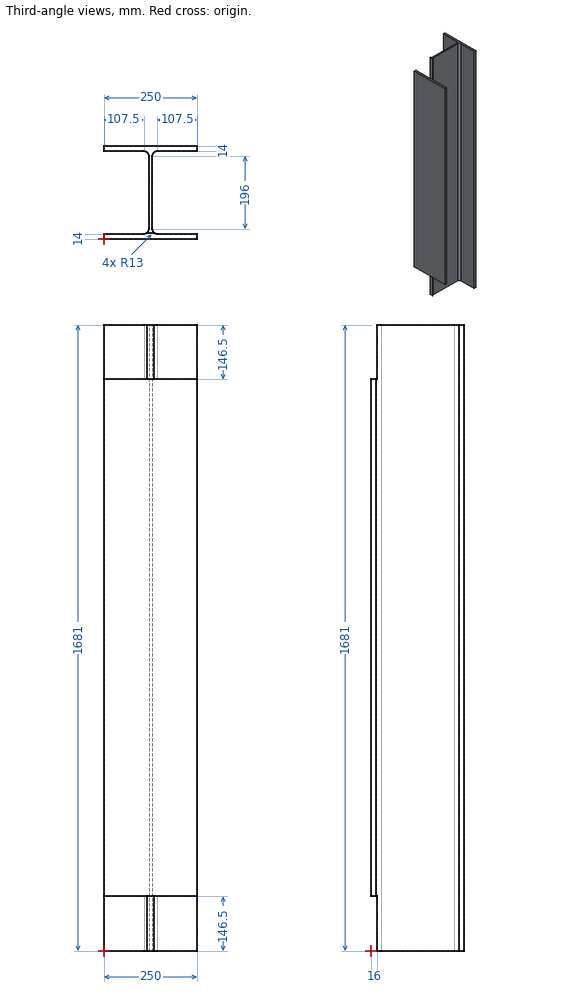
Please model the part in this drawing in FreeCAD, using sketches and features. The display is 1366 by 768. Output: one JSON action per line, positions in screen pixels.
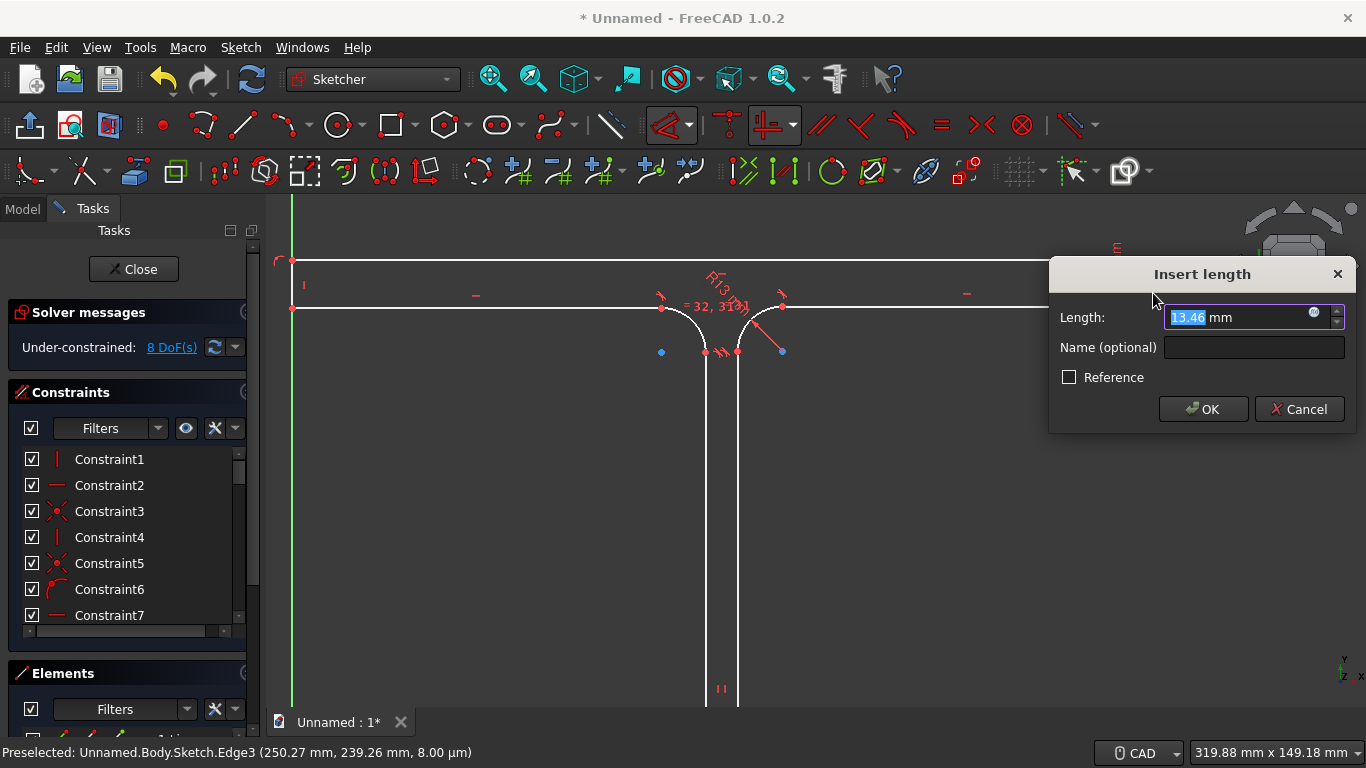
{"action": "type", "text": "14"}
{"action": "key", "text": "Return"}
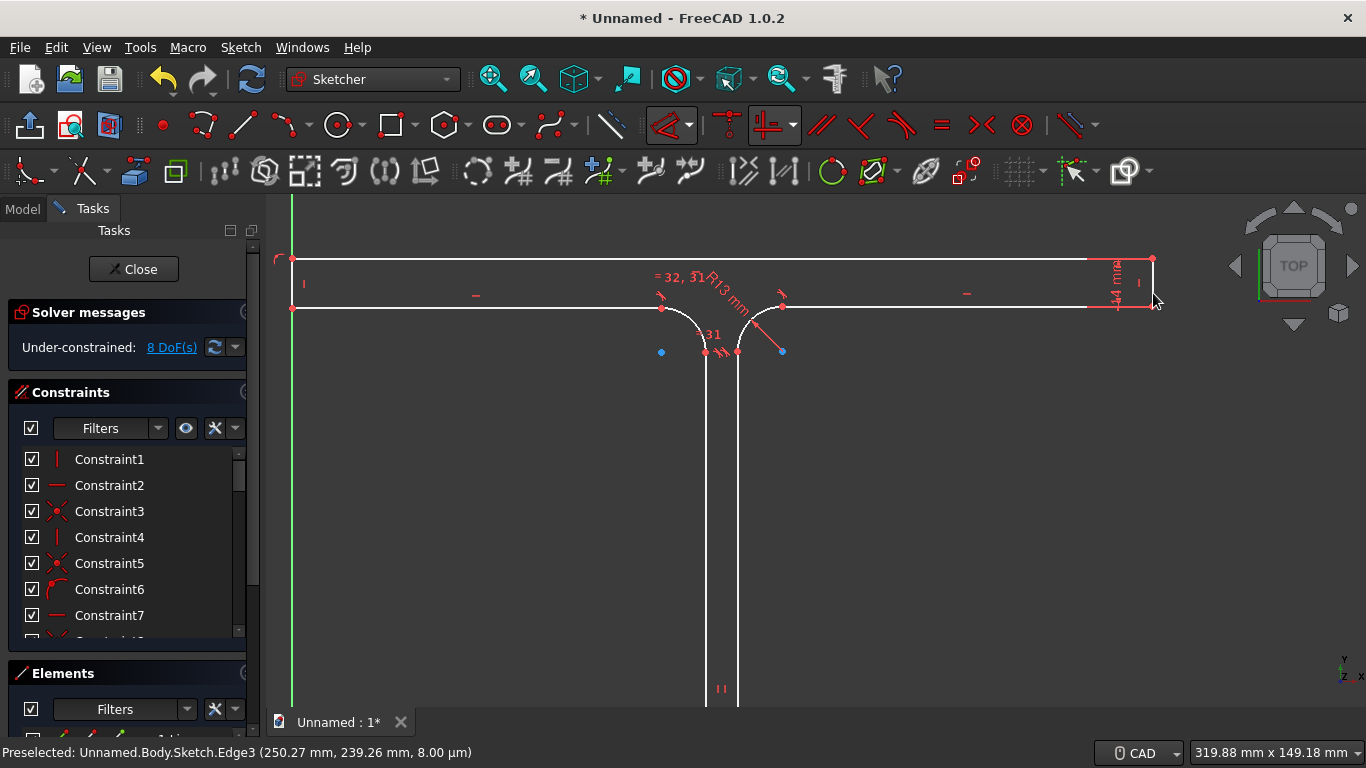
{"action": "scroll", "coordinate": [762, 313], "scroll_direction": "down", "scroll_amount": 5}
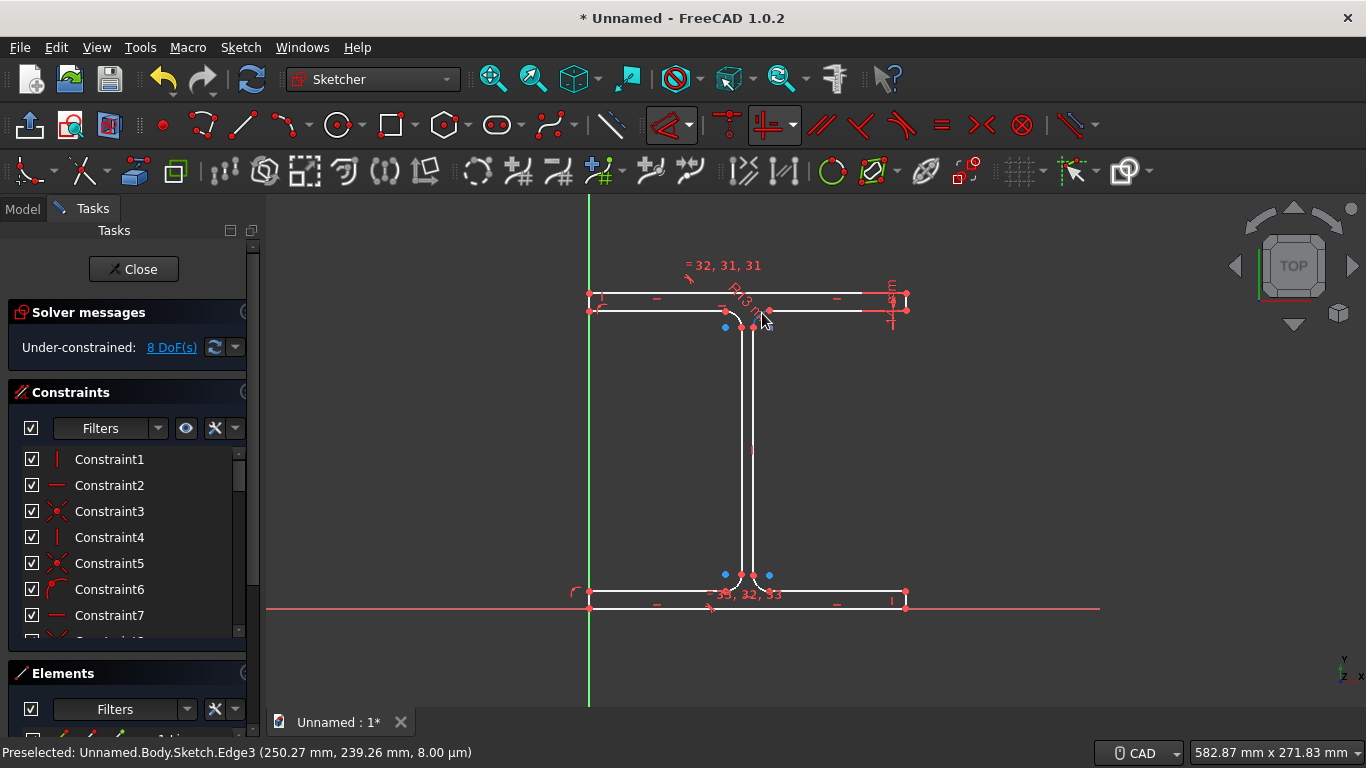
{"action": "scroll", "coordinate": [589, 299], "scroll_direction": "up", "scroll_amount": 5}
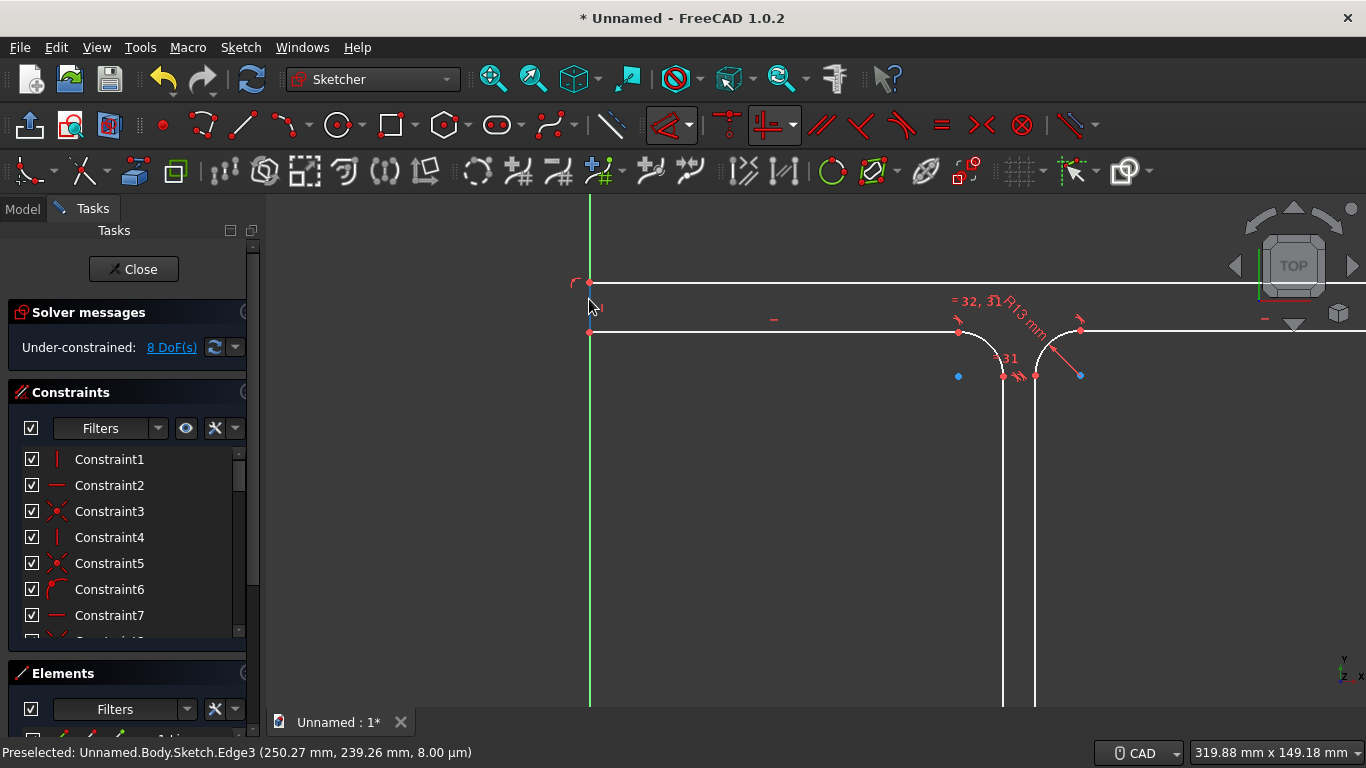
{"action": "left_click", "coordinate": [590, 298]}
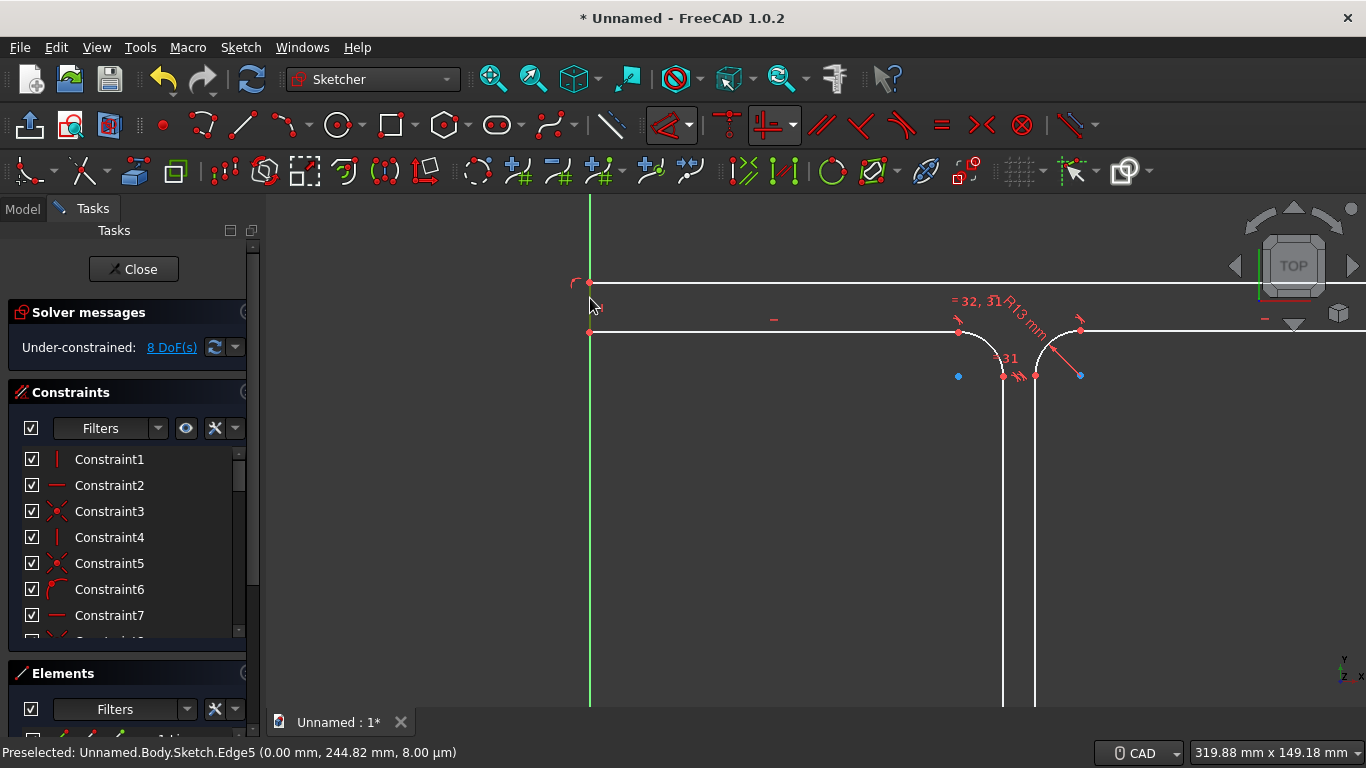
{"action": "key", "text": "i"}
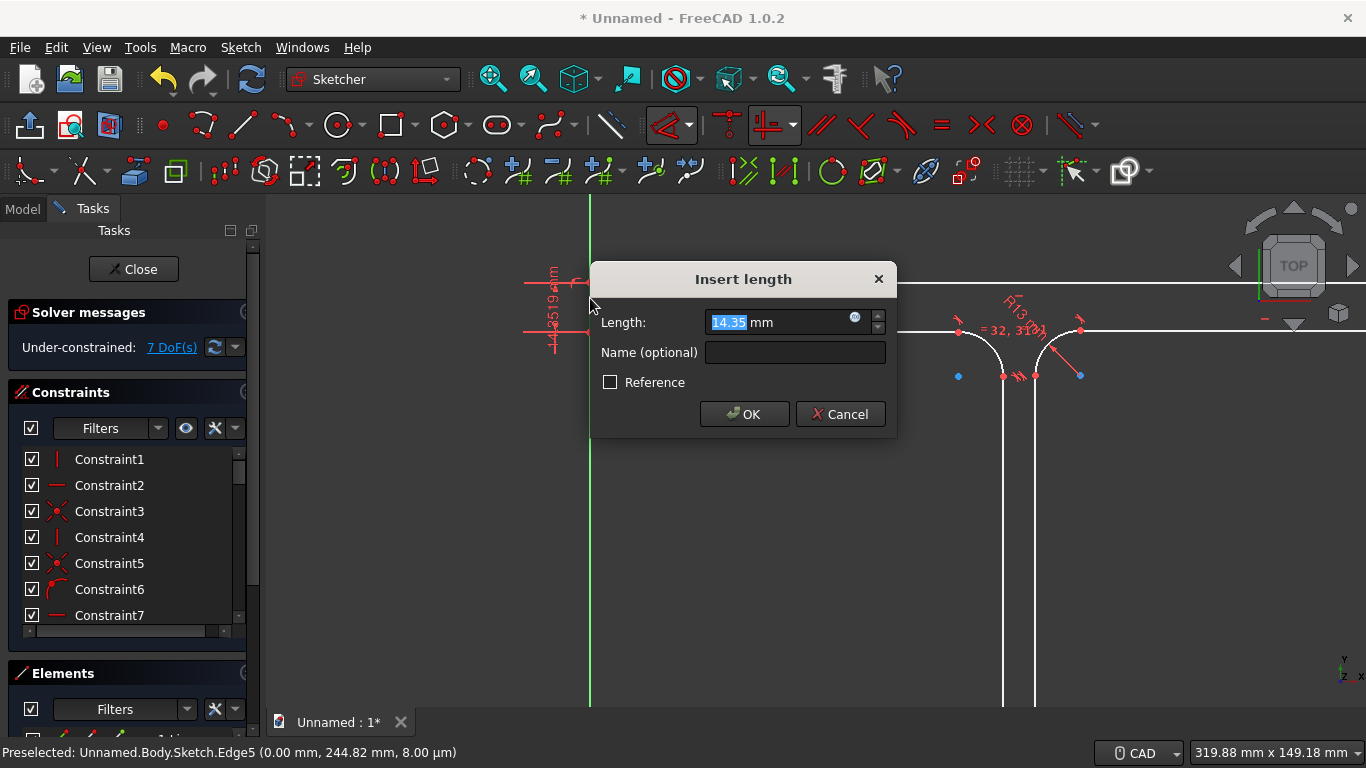
{"action": "type", "text": "14"}
{"action": "key", "text": "Return"}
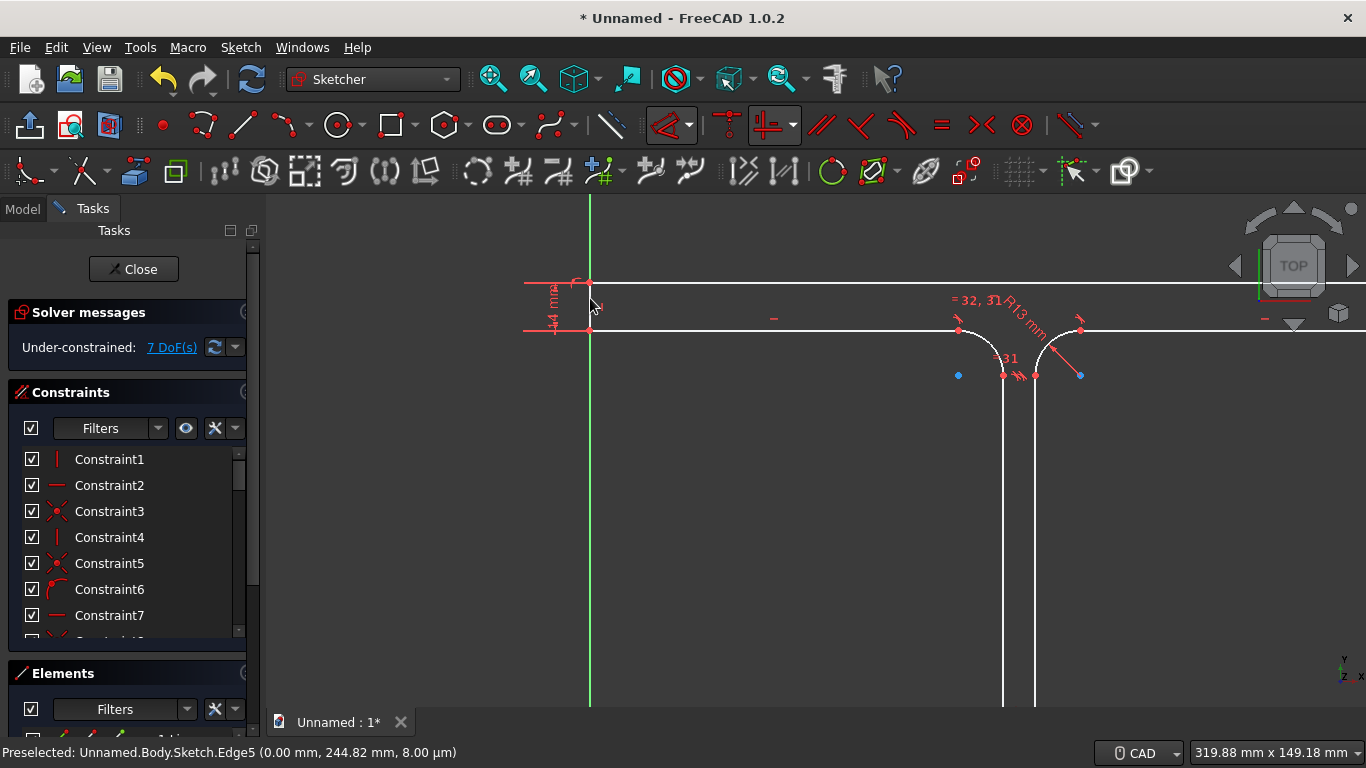
{"action": "scroll", "coordinate": [589, 299], "scroll_direction": "down", "scroll_amount": 5}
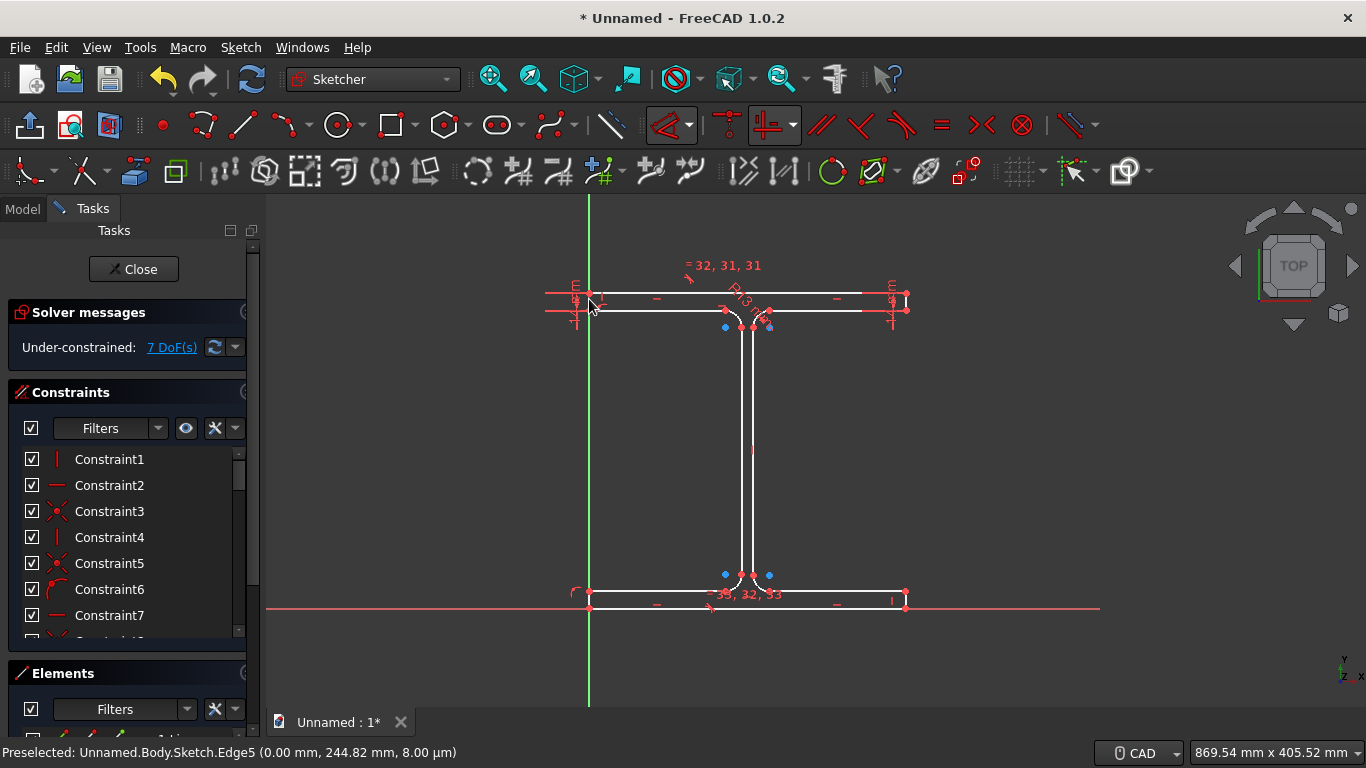
{"action": "scroll", "coordinate": [589, 596], "scroll_direction": "up", "scroll_amount": 5}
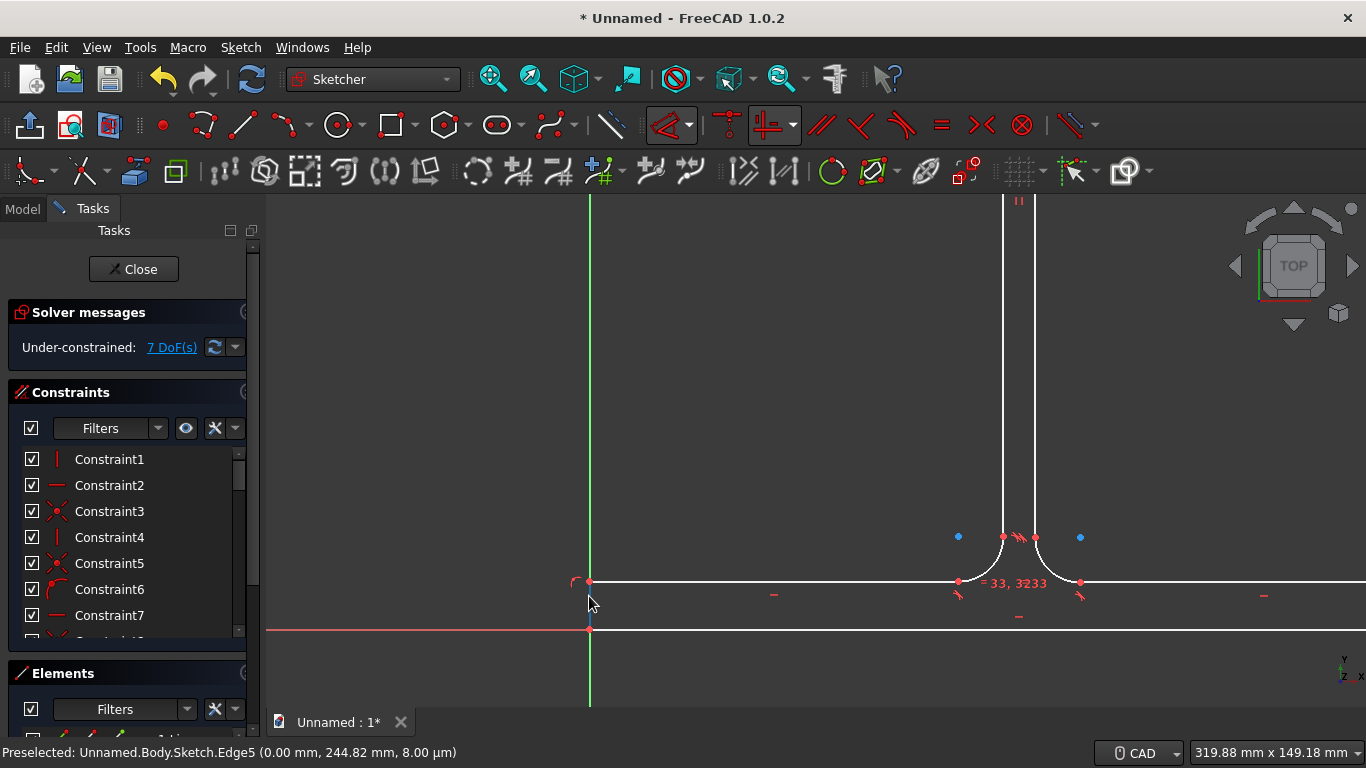
{"action": "left_click", "coordinate": [590, 596]}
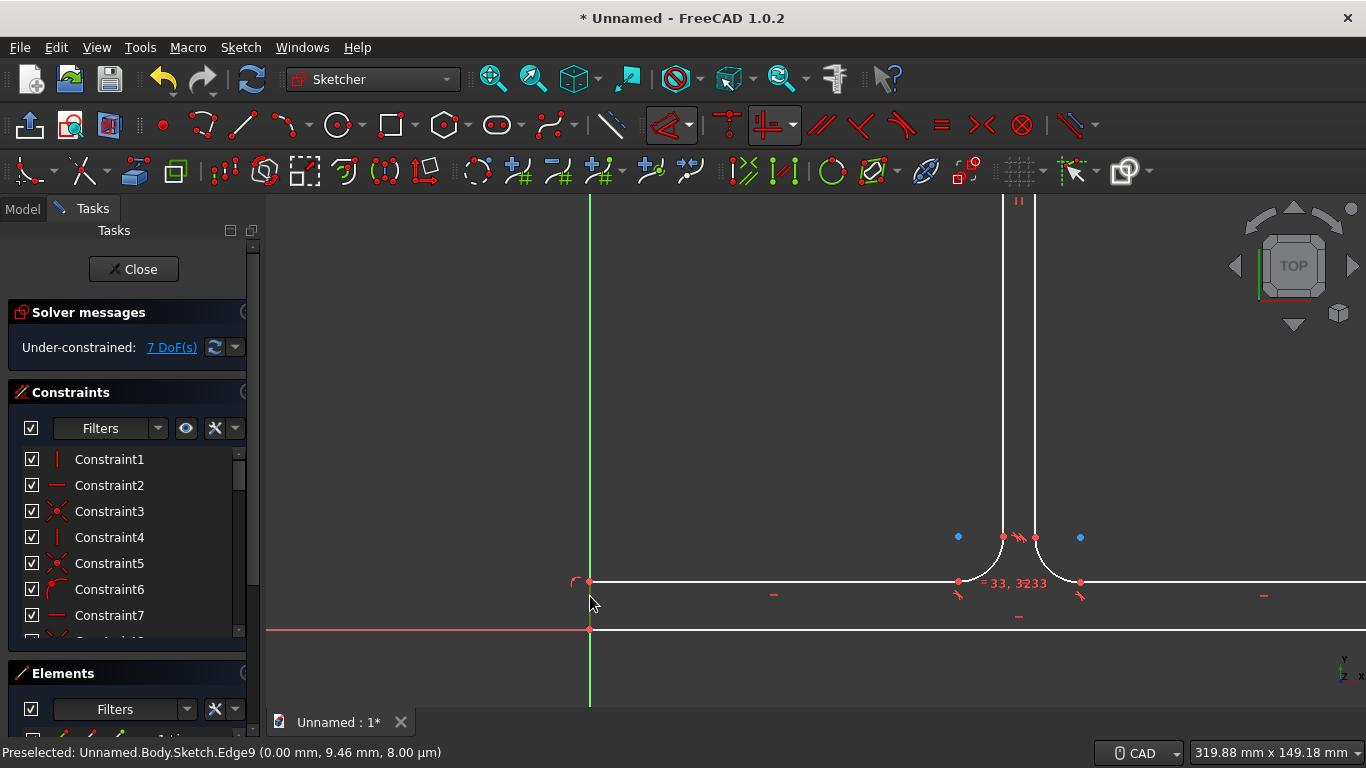
{"action": "left_click", "coordinate": [692, 126]}